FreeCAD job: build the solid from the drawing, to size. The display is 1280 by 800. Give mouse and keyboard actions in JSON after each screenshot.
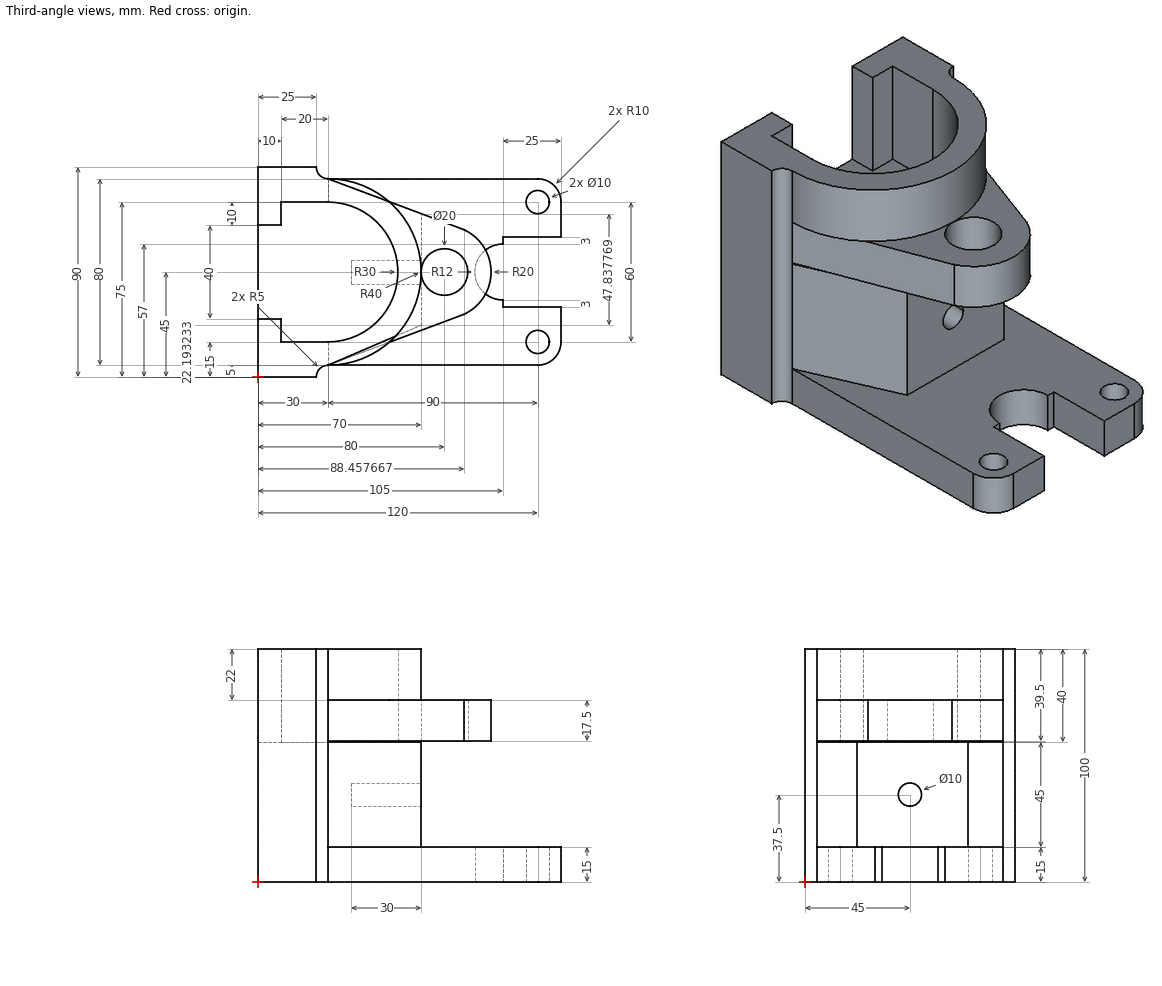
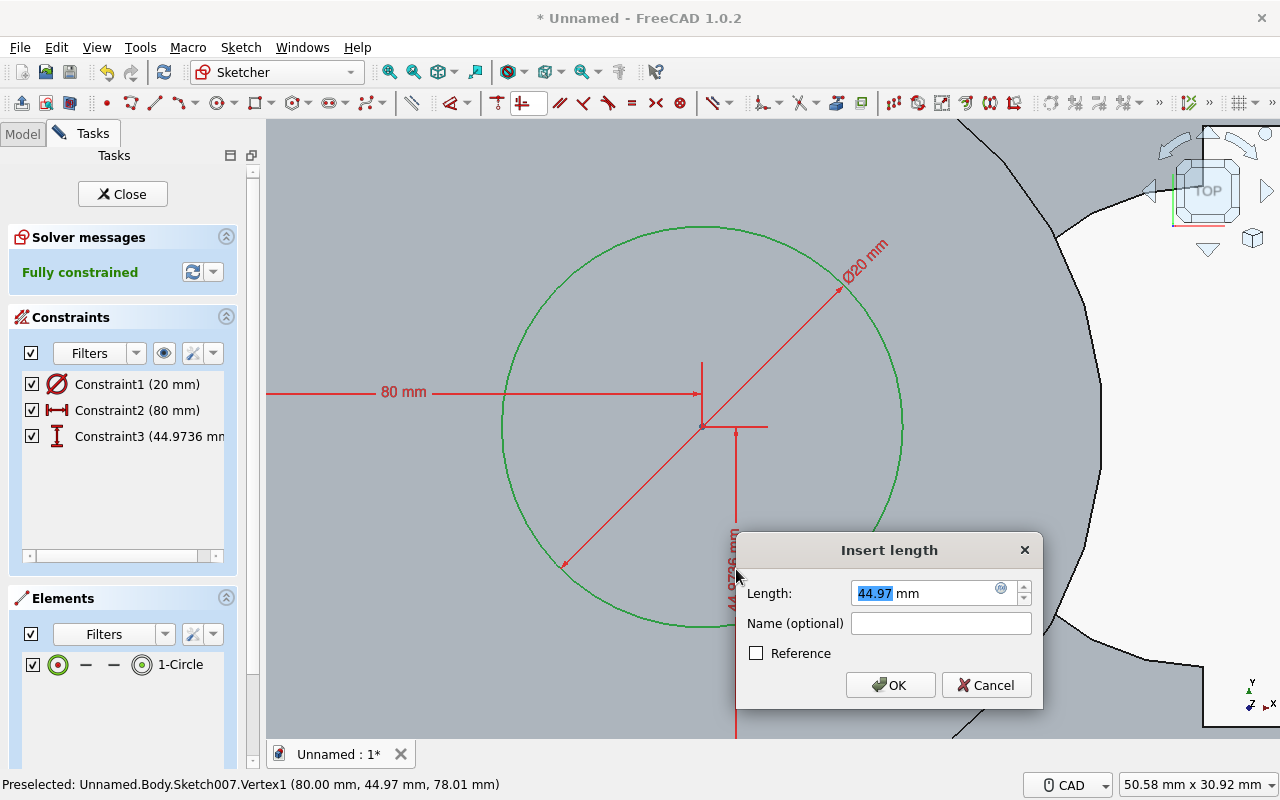
{"action": "type", "text": "45"}
{"action": "key", "text": "Return"}
{"action": "key", "text": "Escape"}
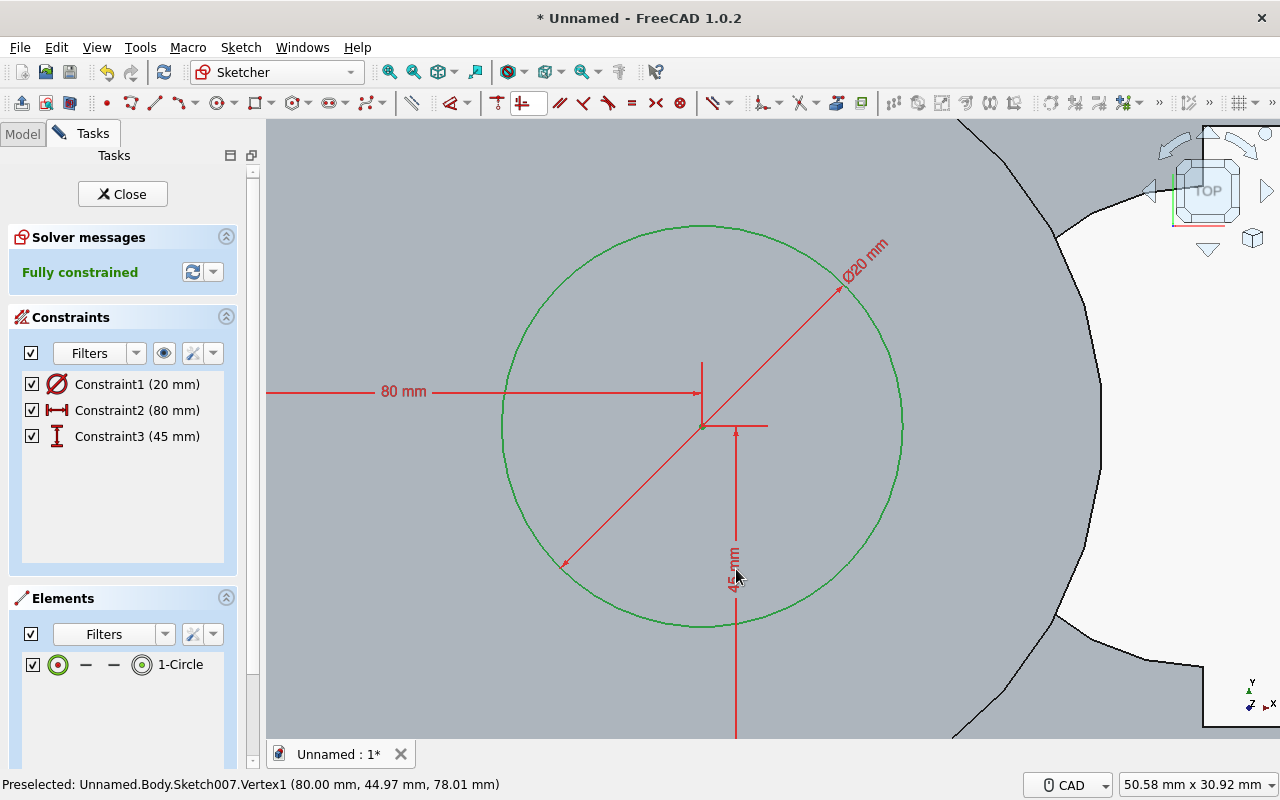
{"action": "left_click", "coordinate": [123, 194]}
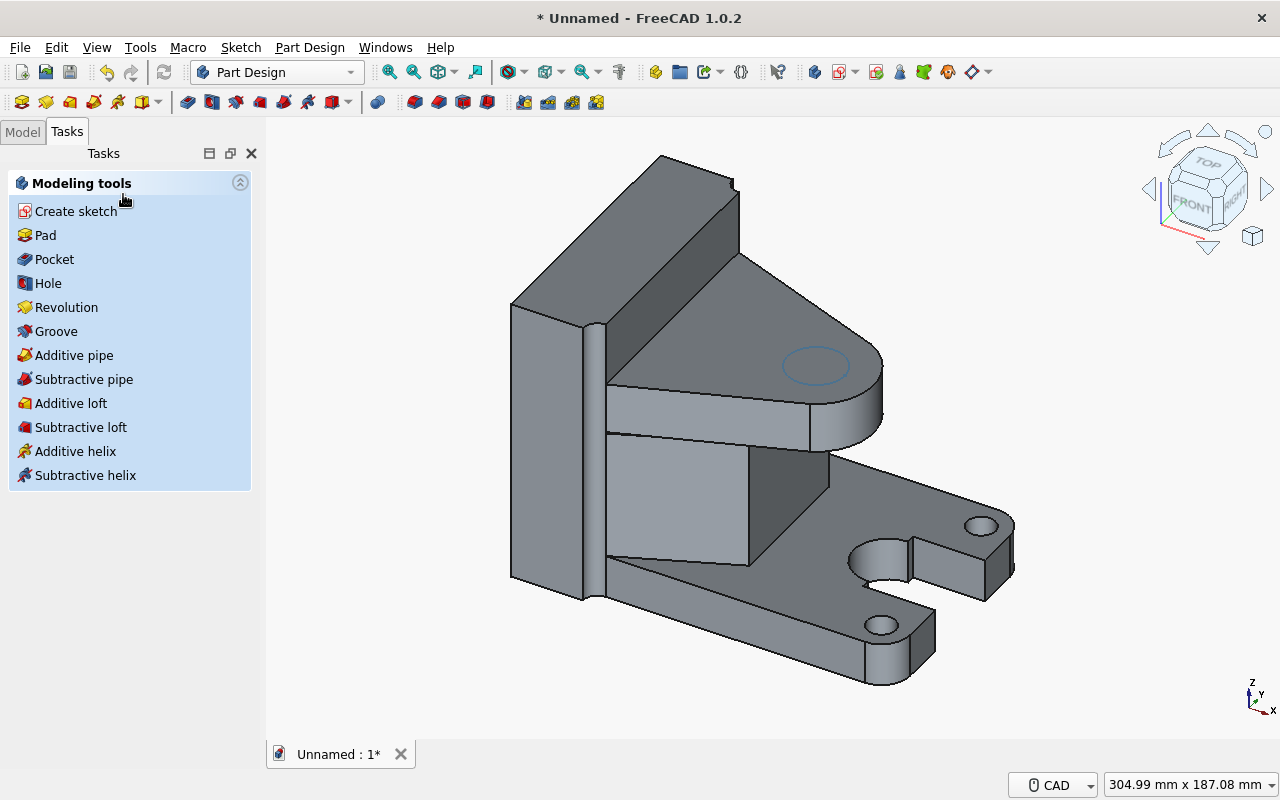
{"action": "left_click", "coordinate": [188, 102]}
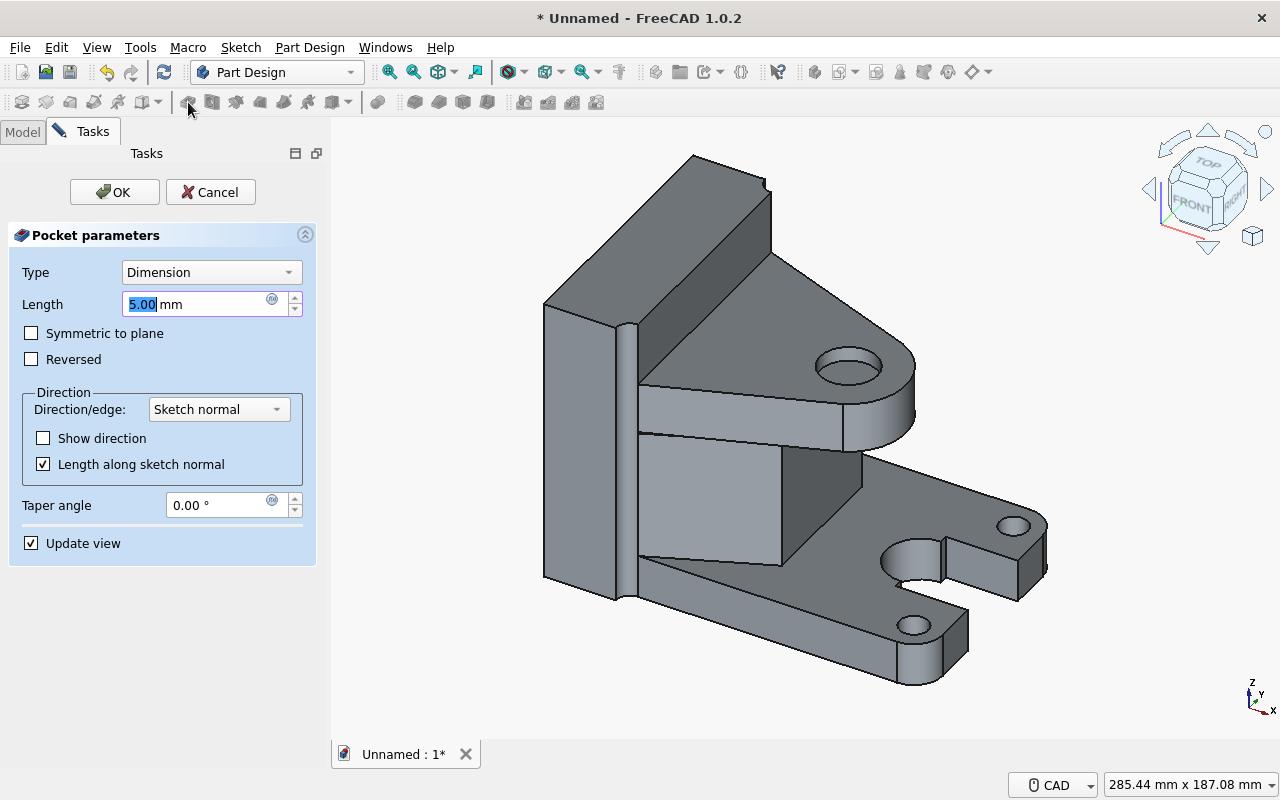
{"action": "type", "text": "17.5"}
{"action": "key", "text": "Tab"}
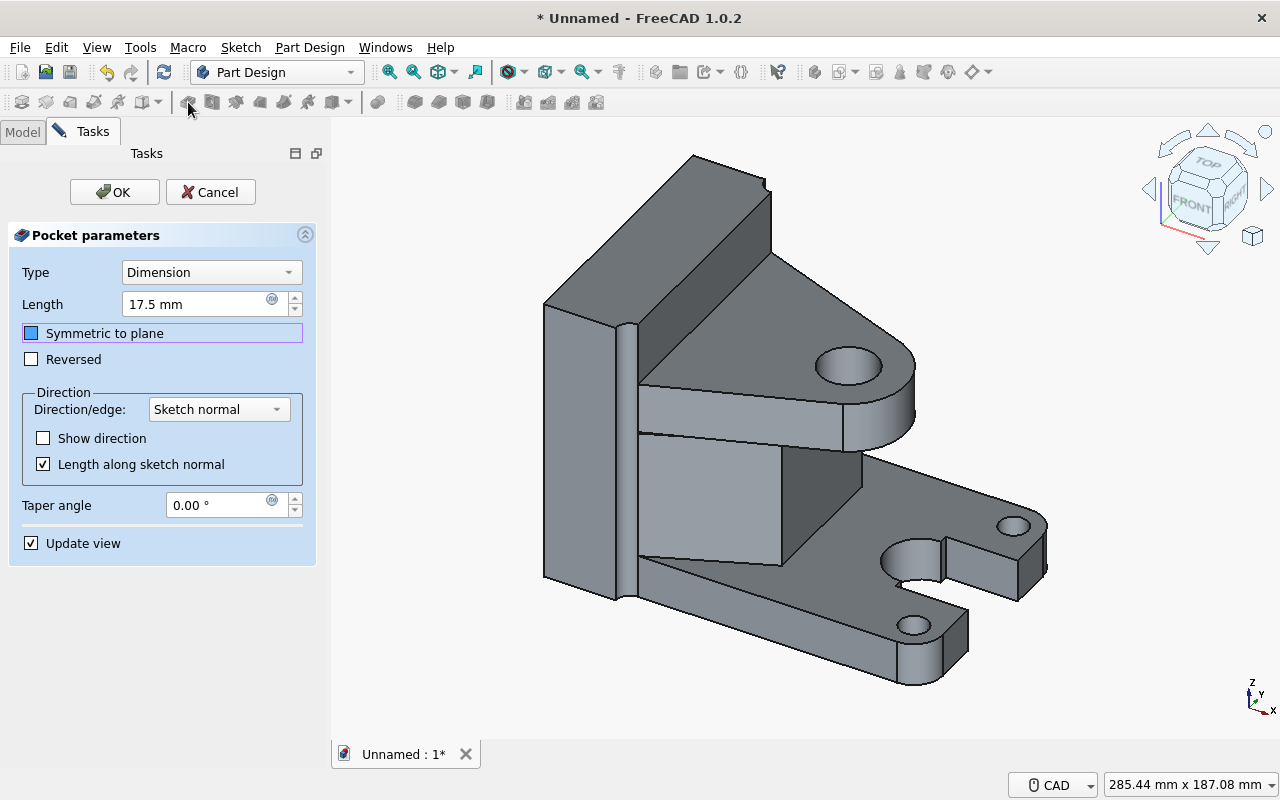
{"action": "left_click", "coordinate": [115, 192]}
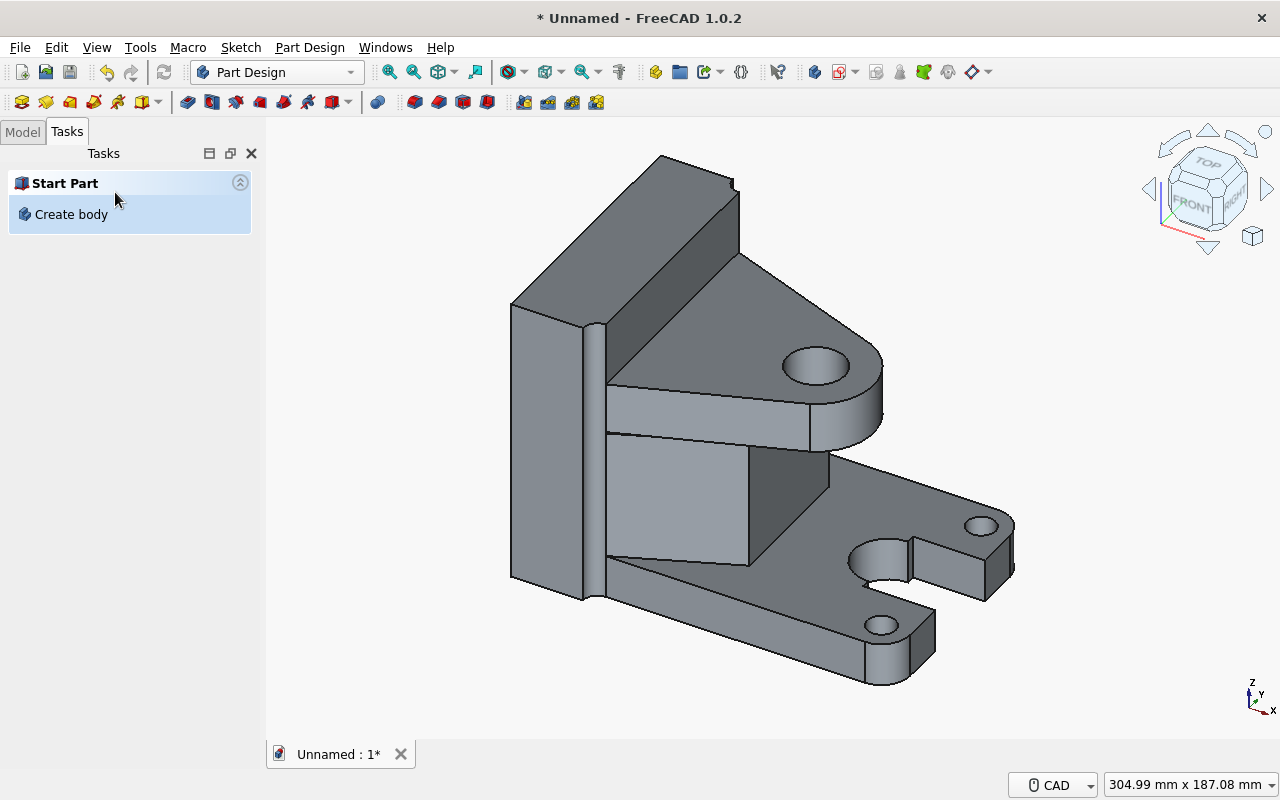
{"action": "left_click", "coordinate": [789, 464]}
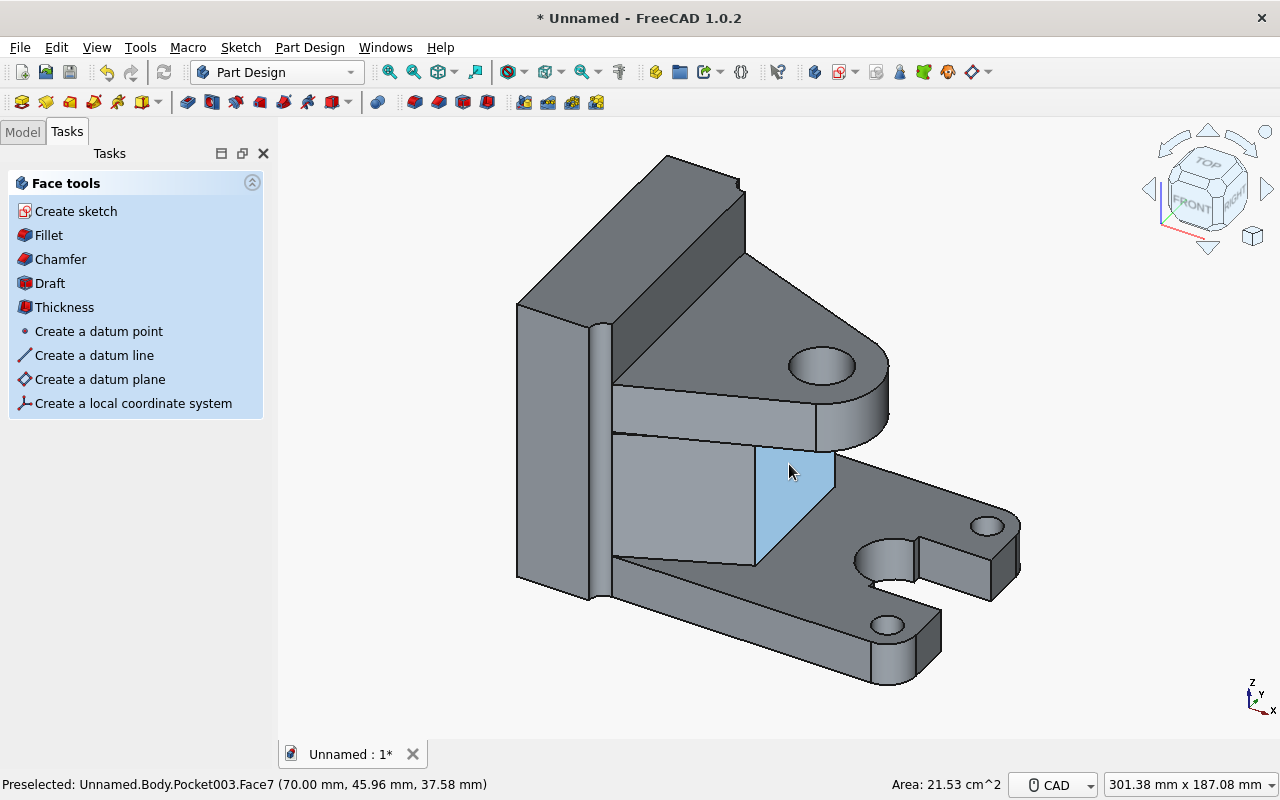
{"action": "left_click", "coordinate": [840, 72]}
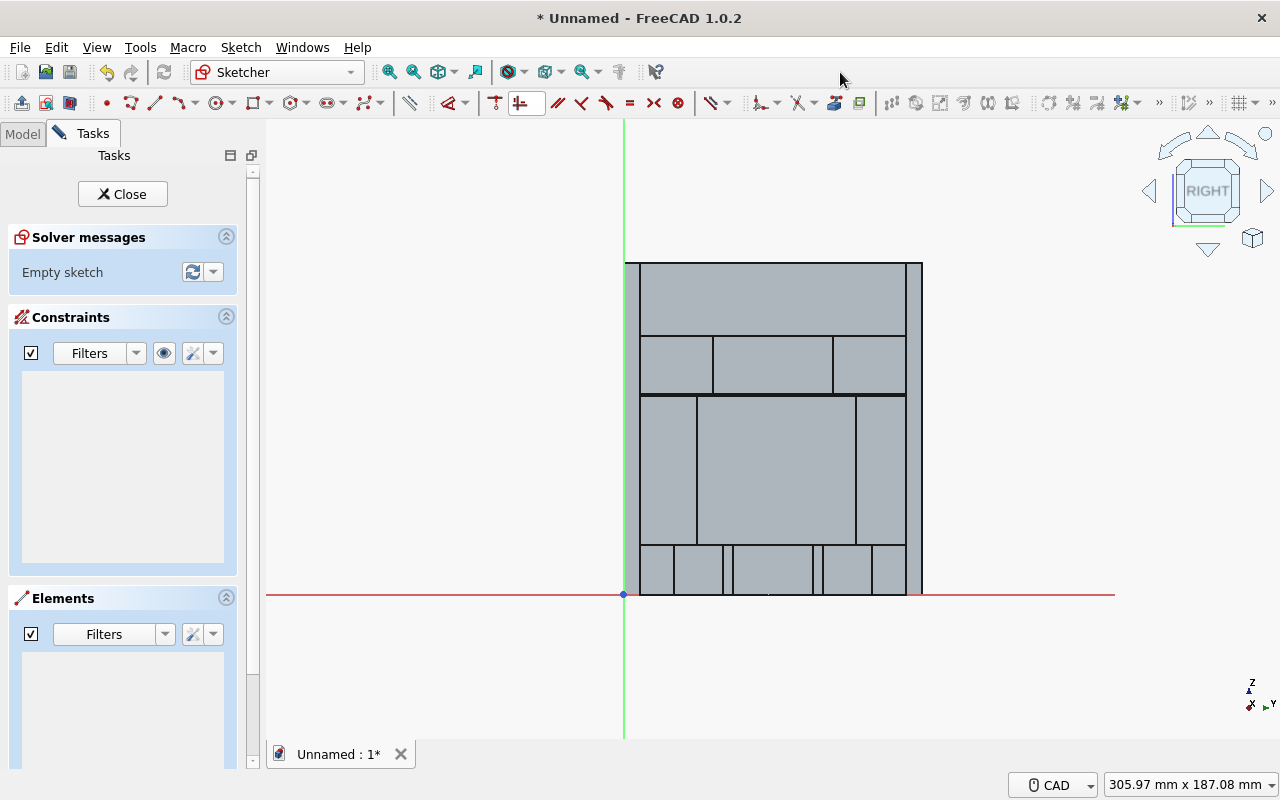
{"action": "key", "text": "q s"}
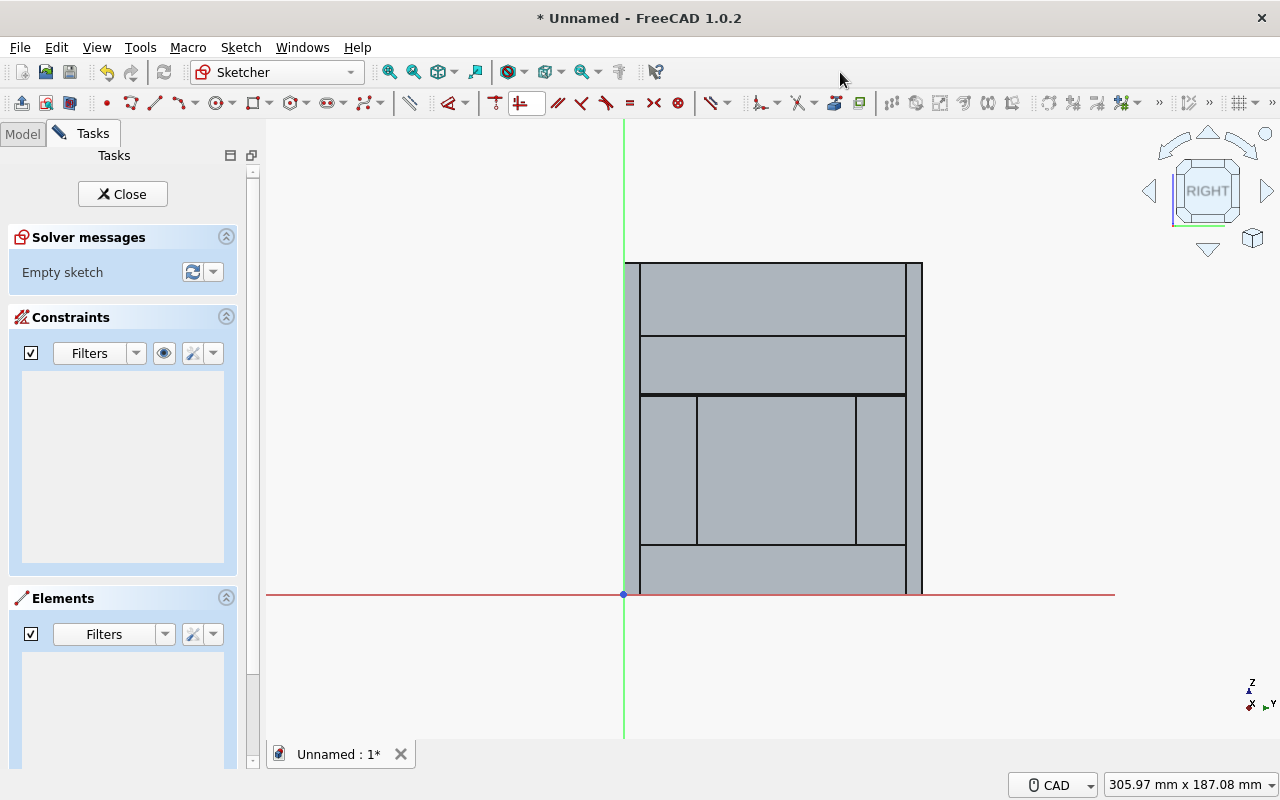
{"action": "scroll", "coordinate": [780, 475], "scroll_direction": "up", "scroll_amount": 12}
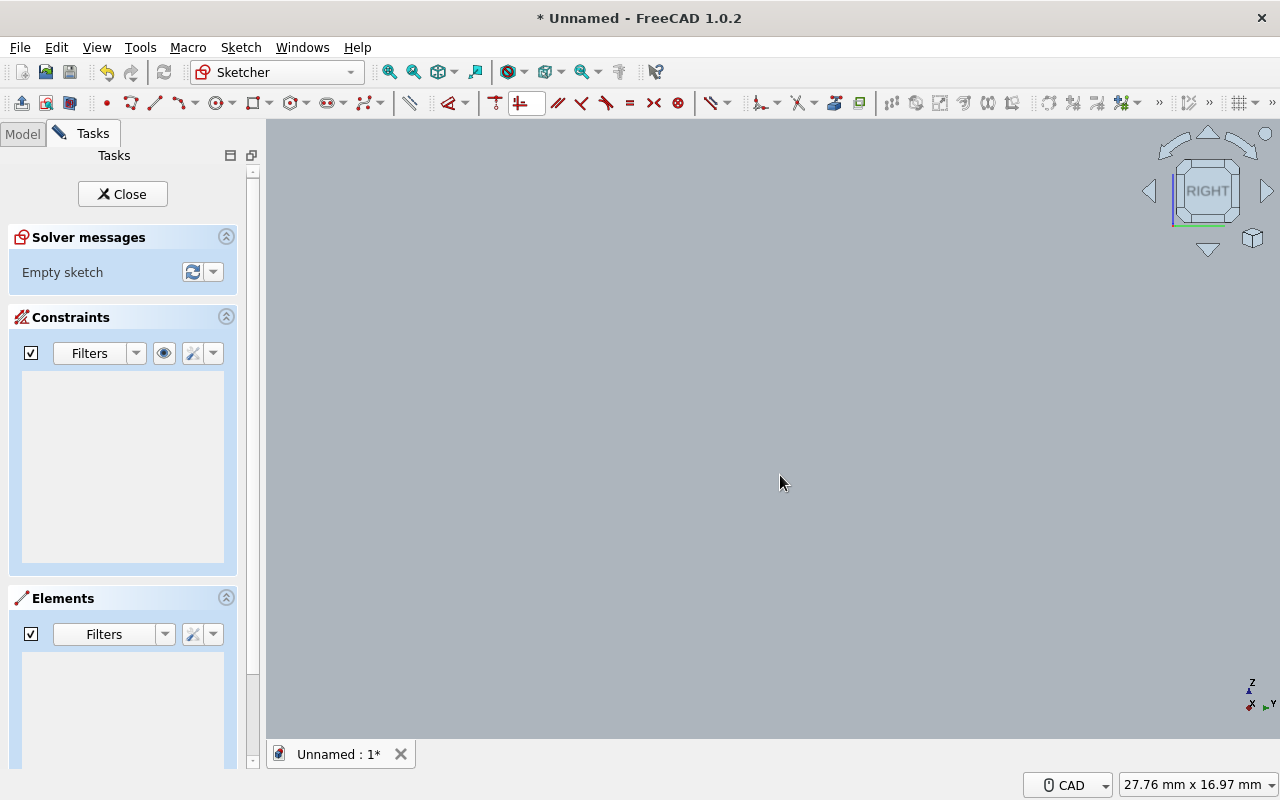
{"action": "left_click", "coordinate": [216, 104]}